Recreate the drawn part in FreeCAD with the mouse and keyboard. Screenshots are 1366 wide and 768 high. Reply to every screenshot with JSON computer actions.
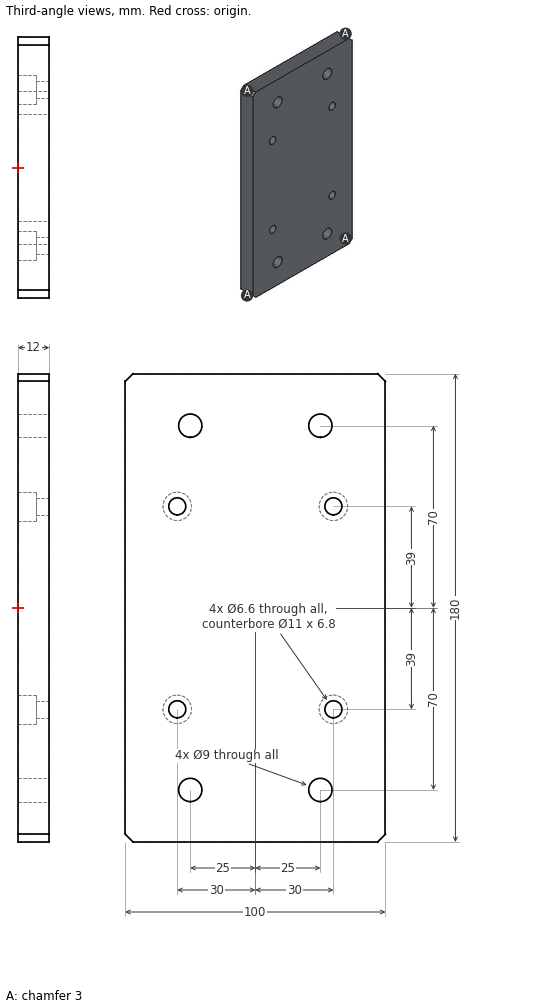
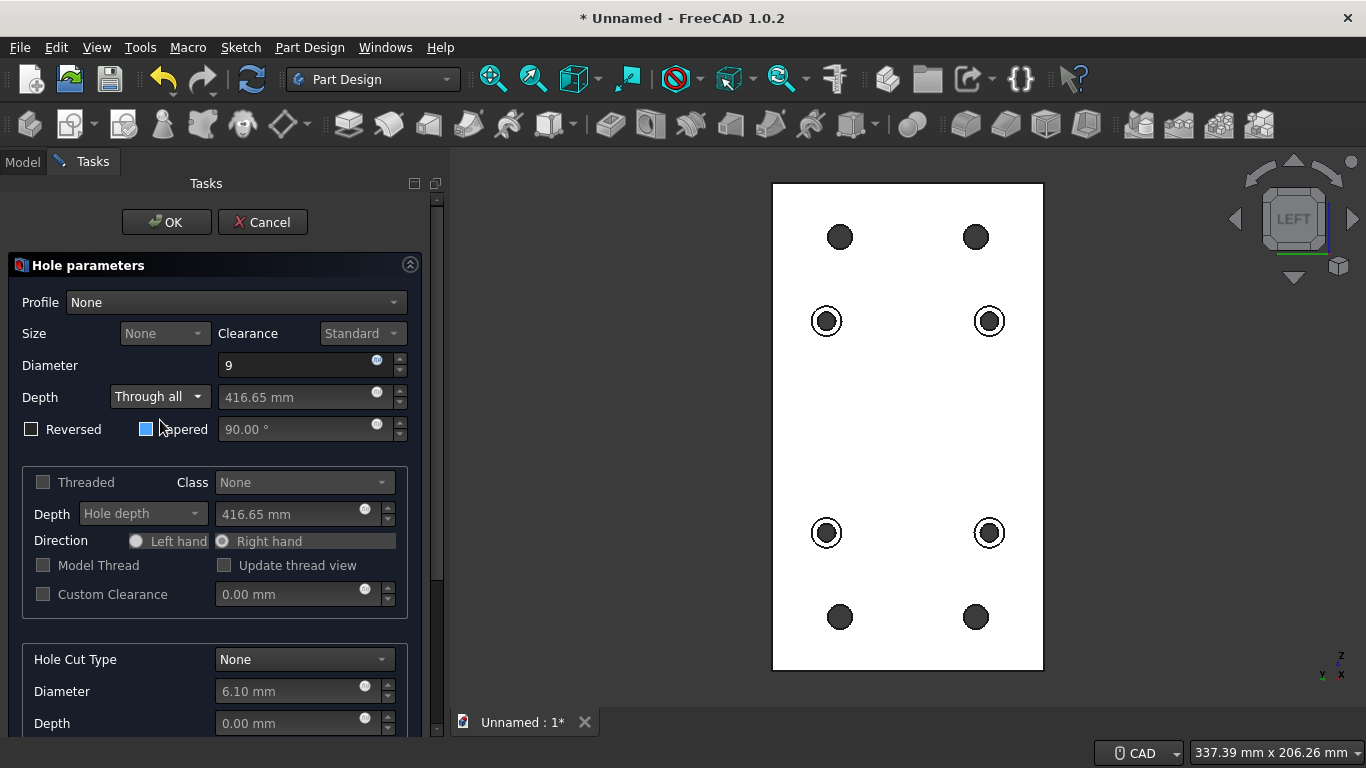
{"action": "left_click", "coordinate": [167, 222]}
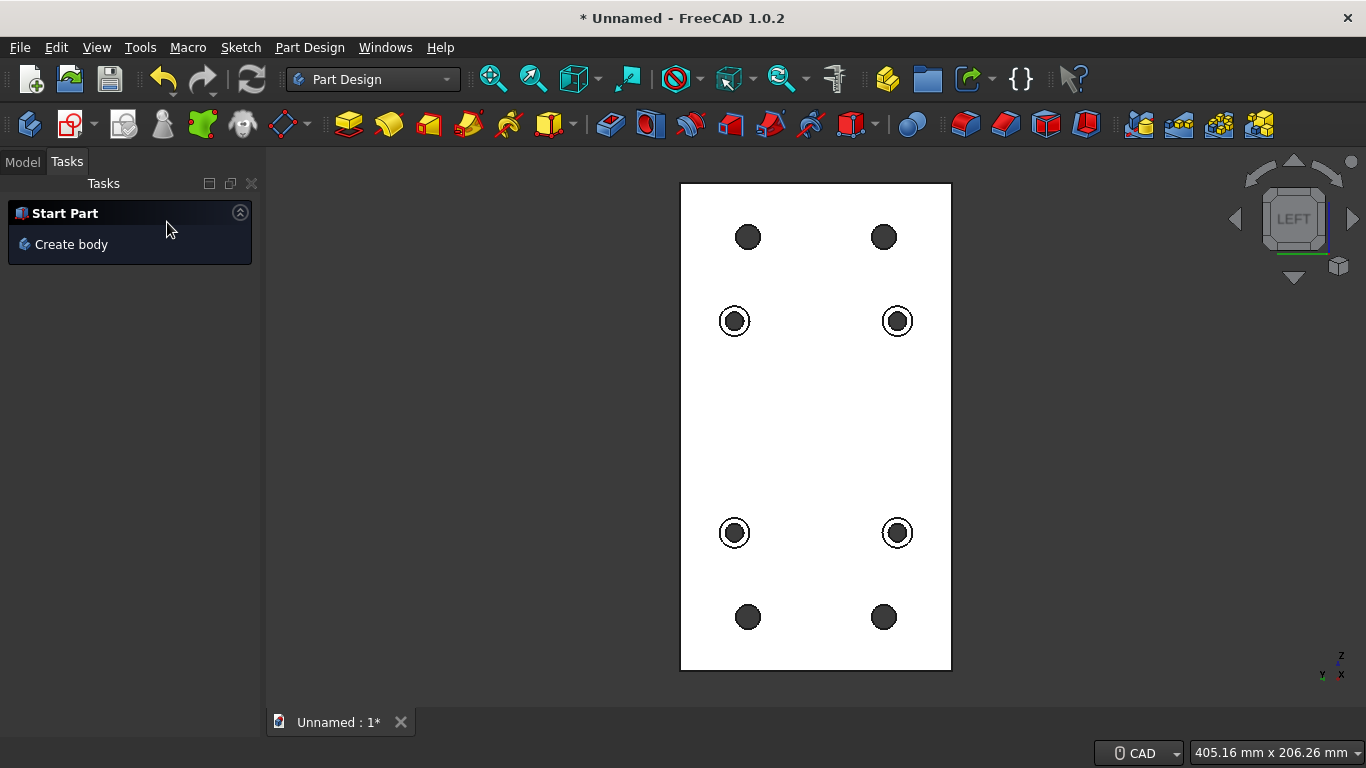
{"action": "key", "text": "0"}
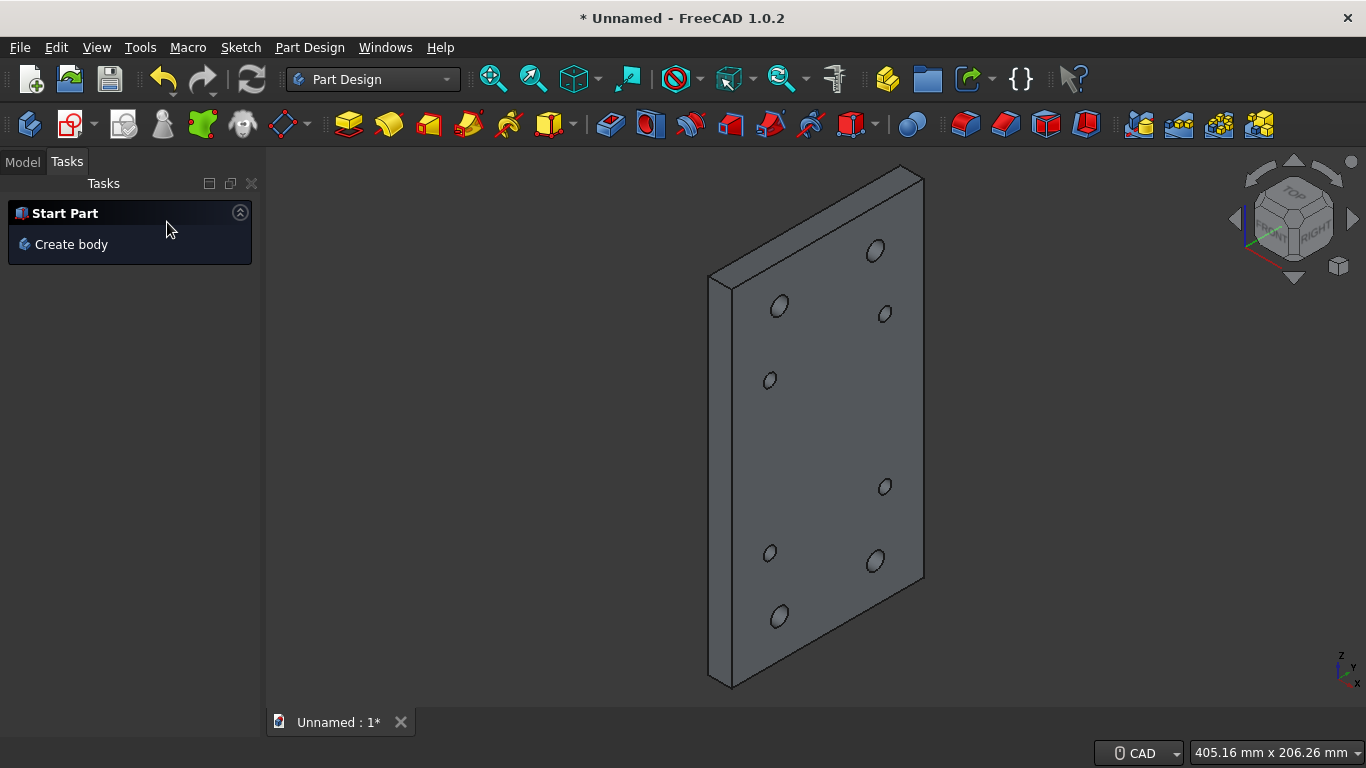
{"action": "left_click", "coordinate": [720, 282]}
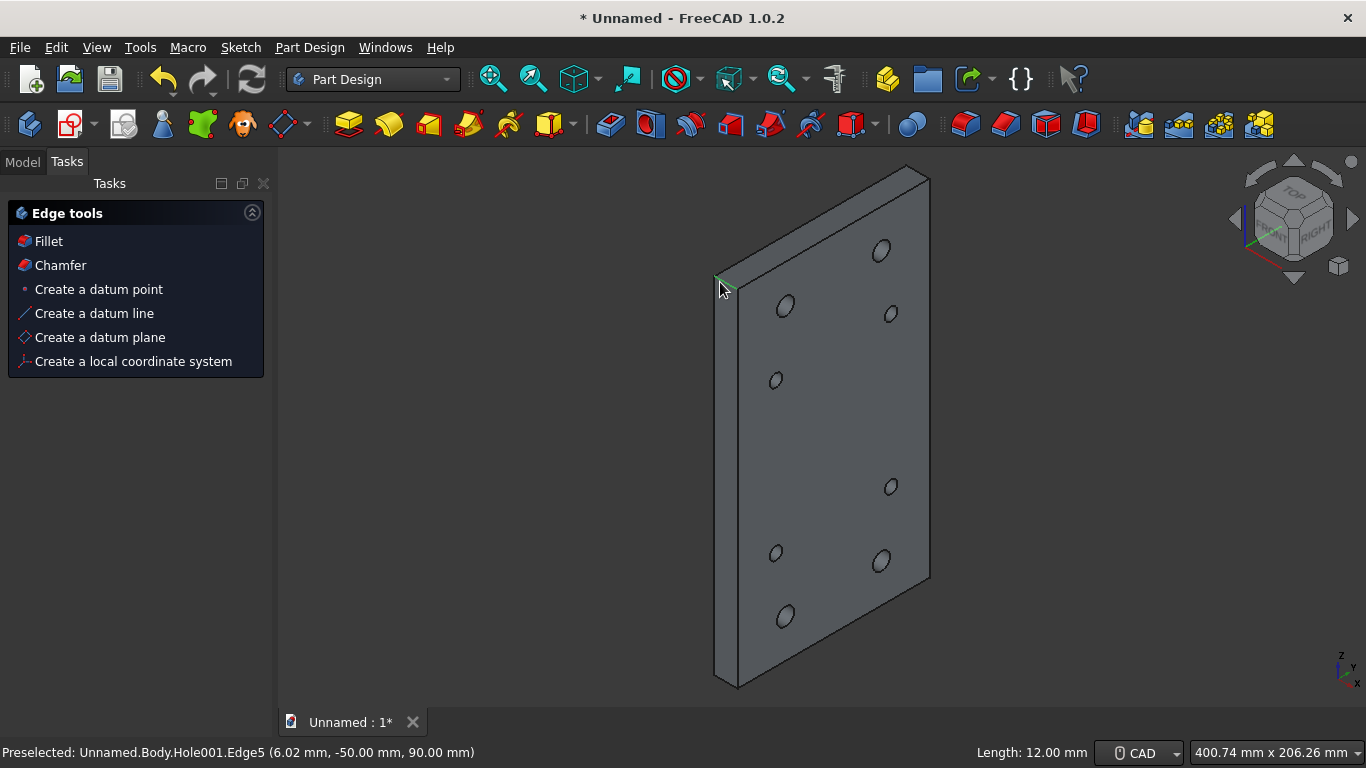
{"action": "key", "text": "2"}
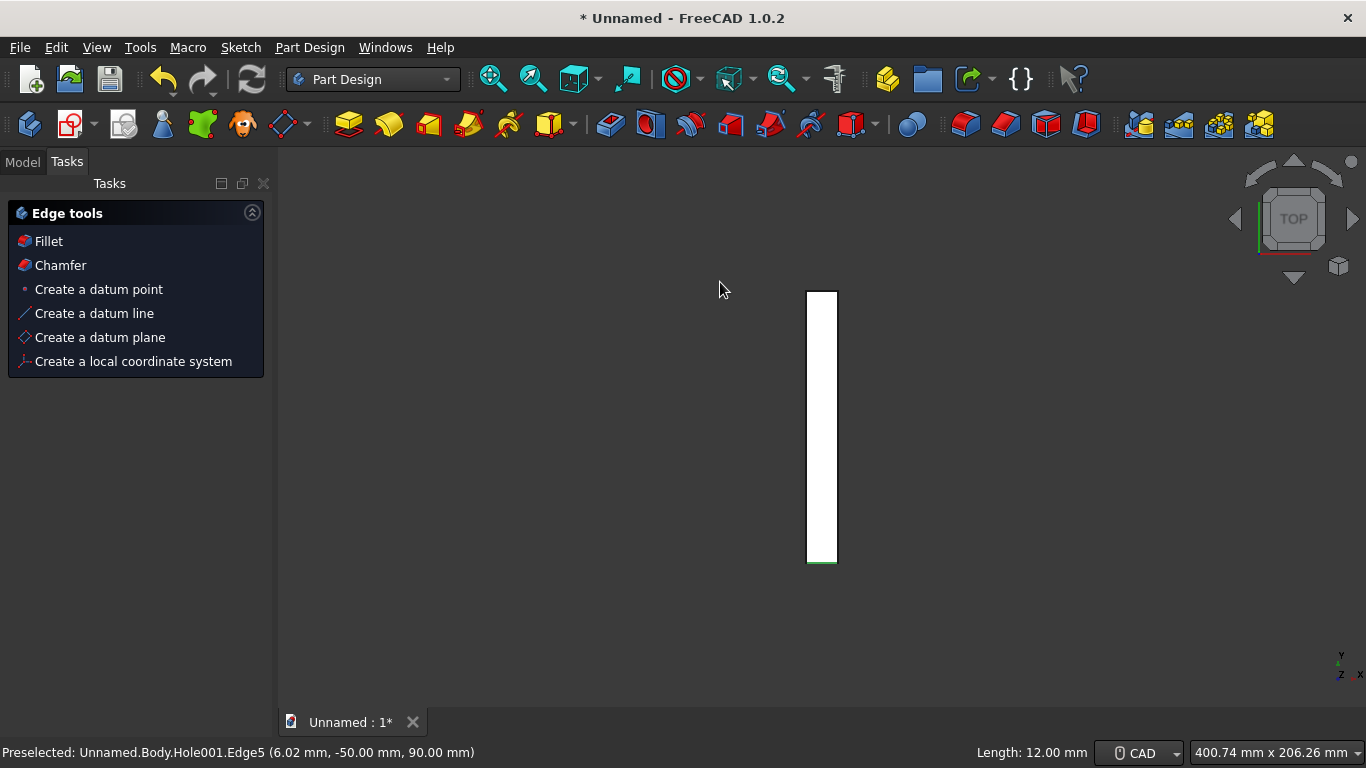
{"action": "left_click", "coordinate": [822, 290], "text": "ctrl"}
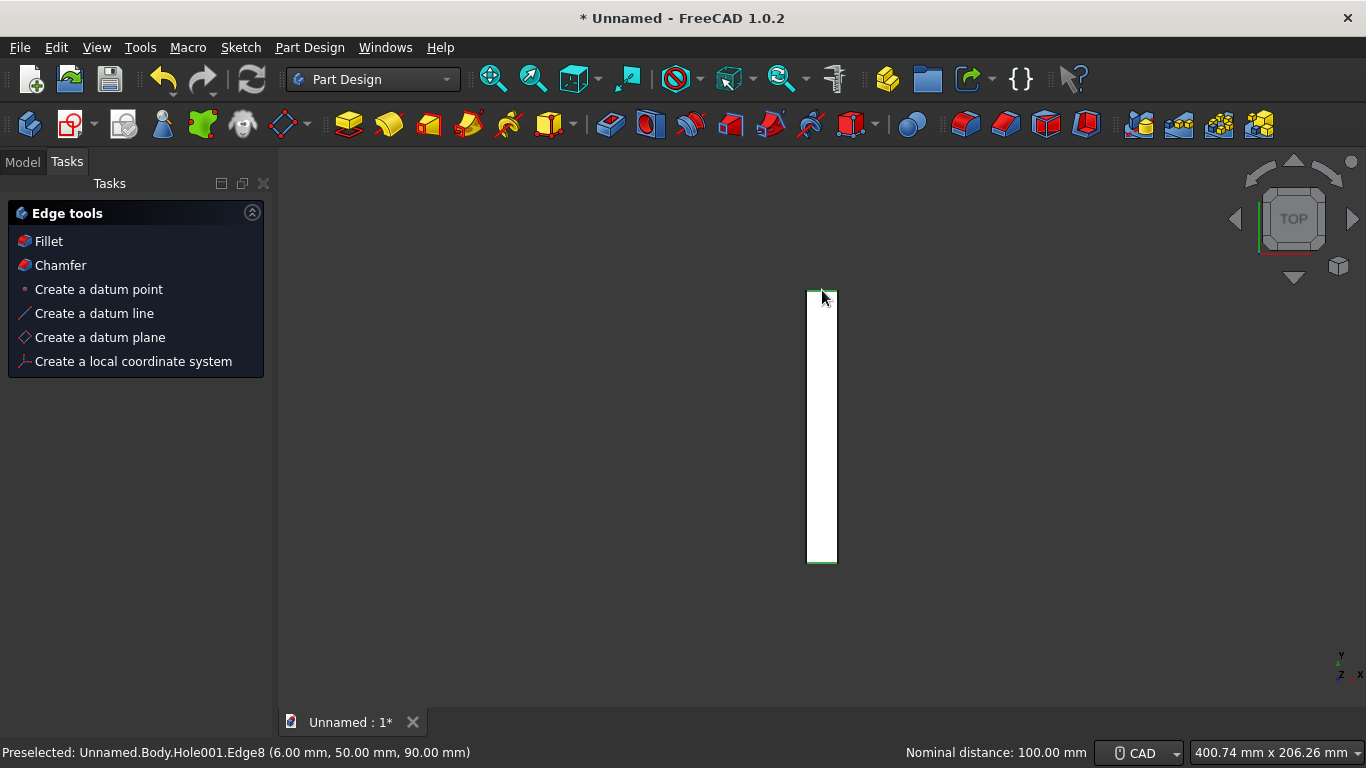
{"action": "key", "text": "1"}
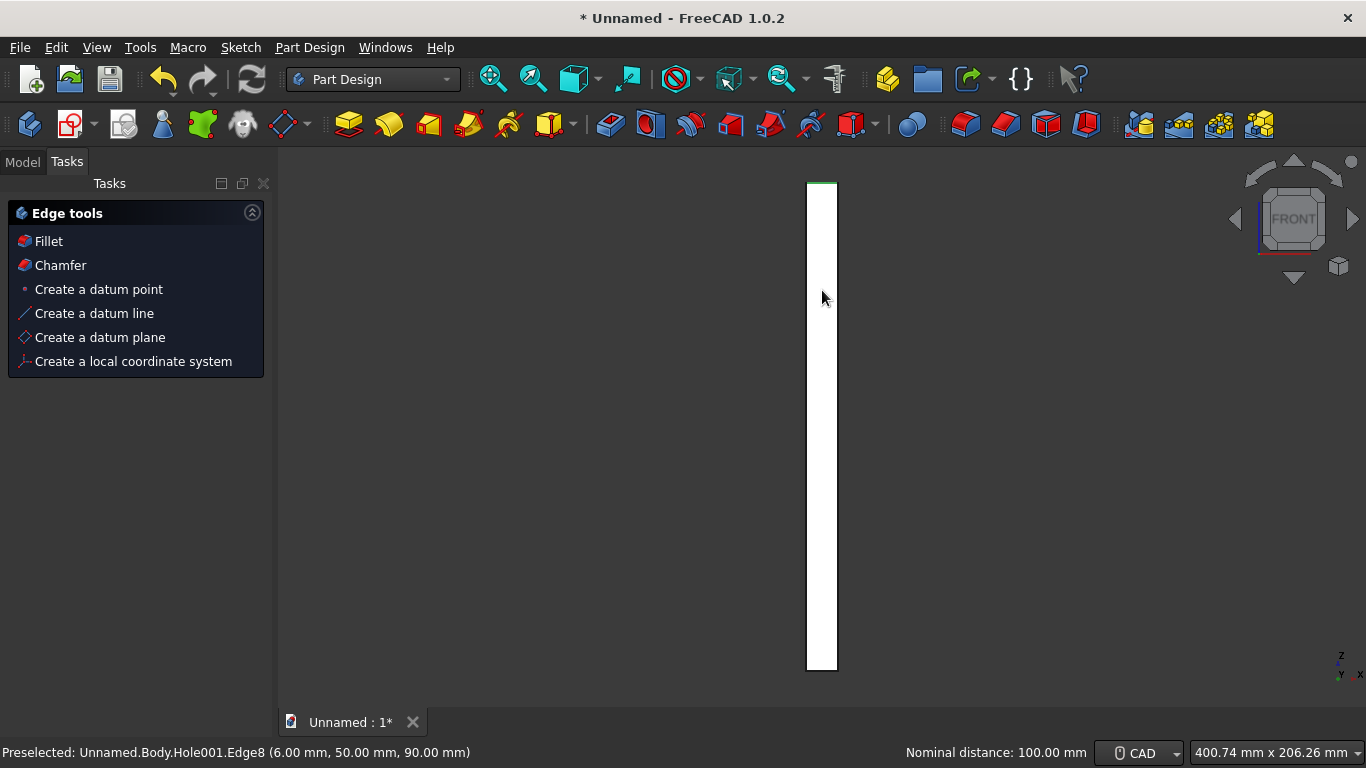
{"action": "left_click", "coordinate": [822, 670], "text": "ctrl"}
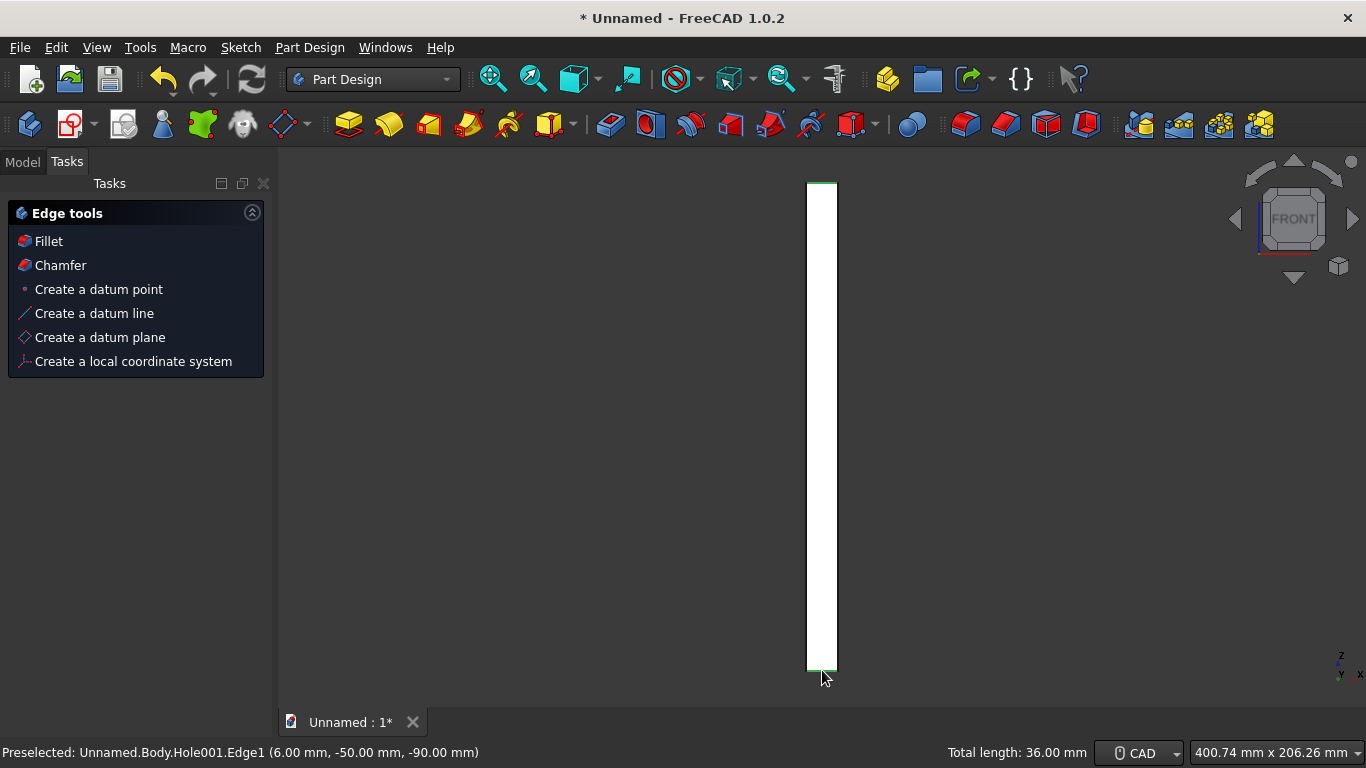
{"action": "key", "text": "3"}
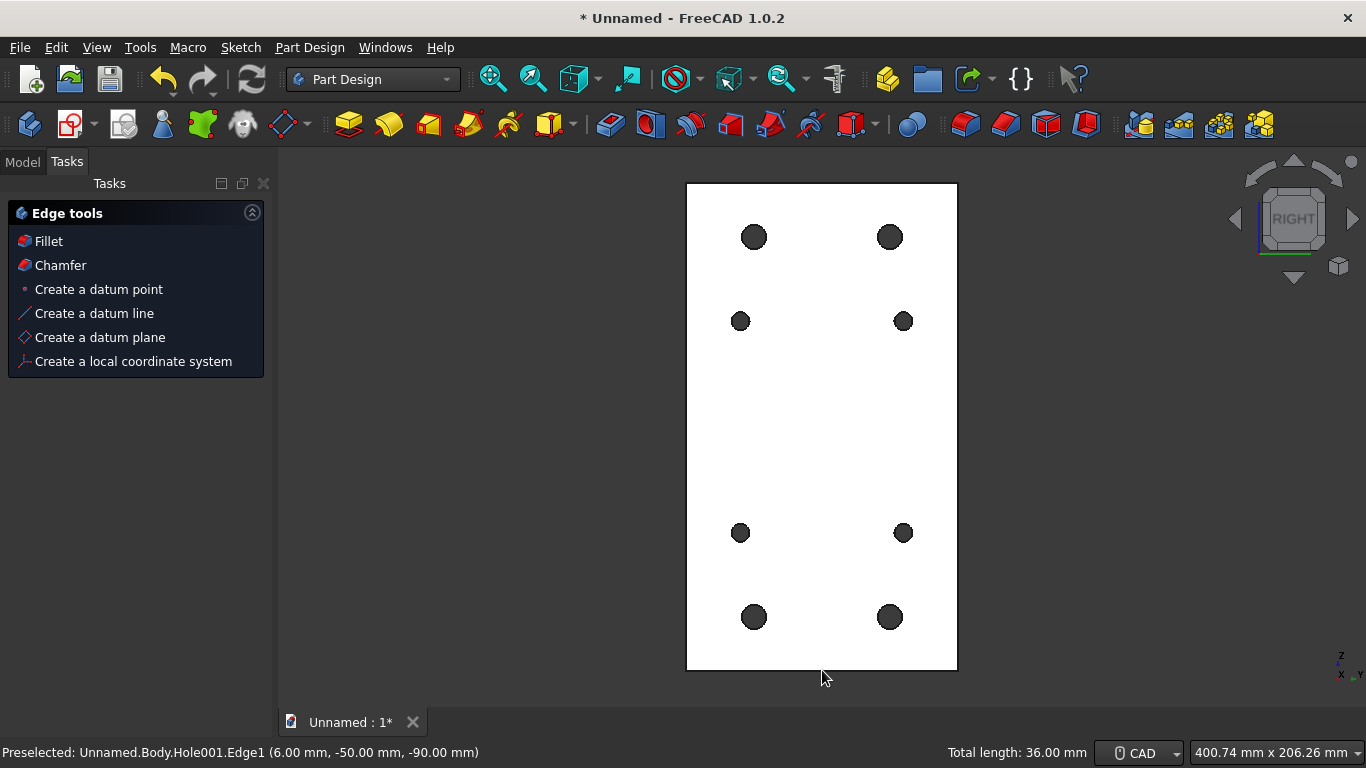
{"action": "key", "text": "5"}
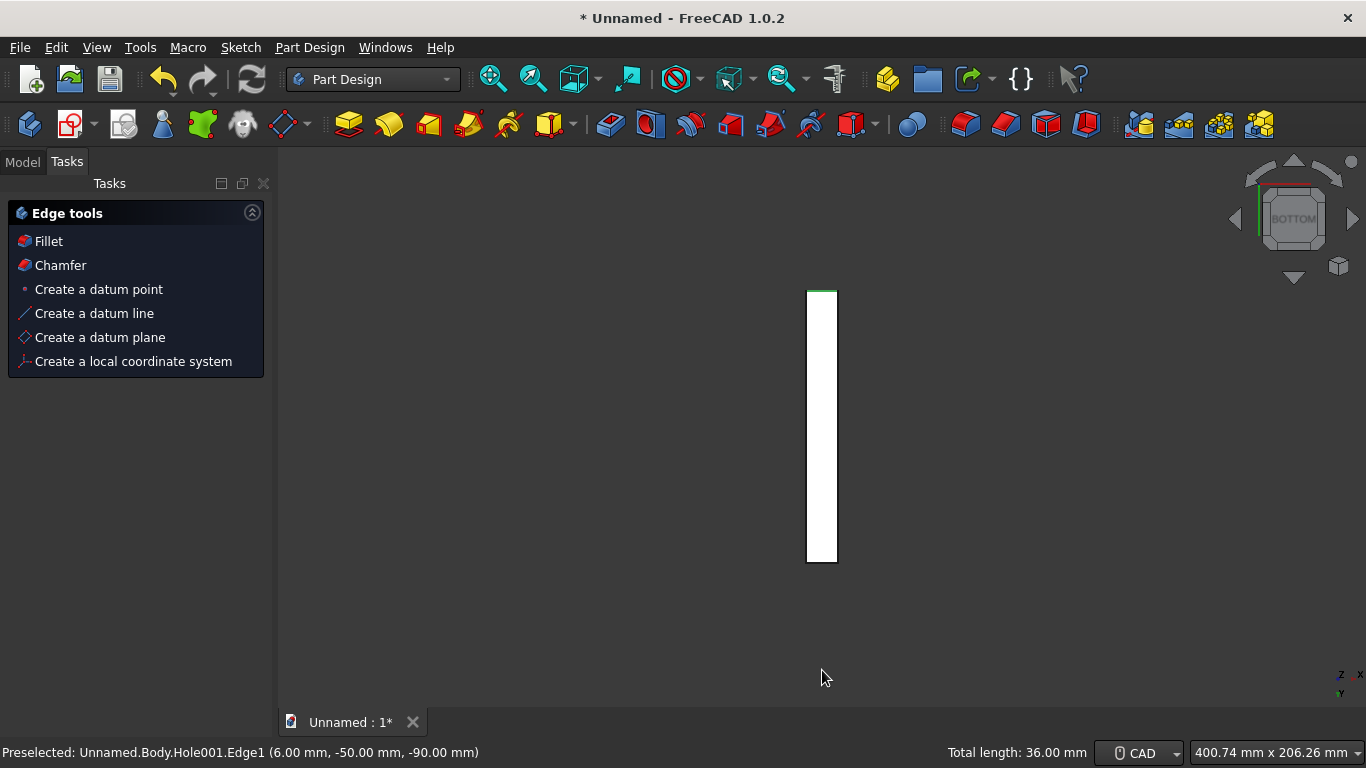
{"action": "left_click", "coordinate": [822, 562], "text": "ctrl"}